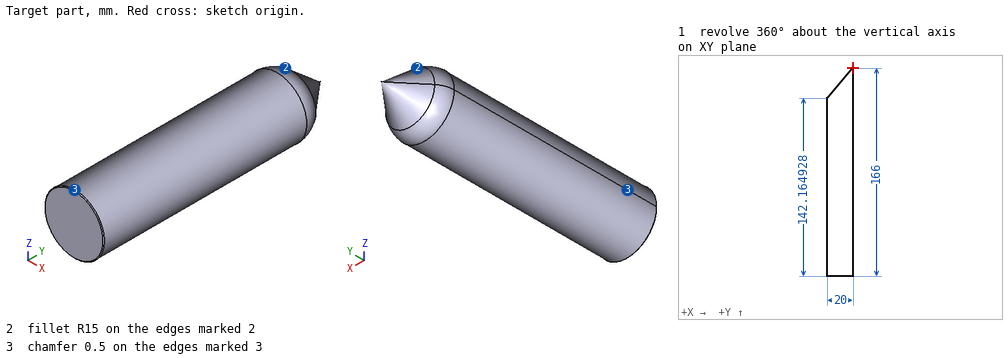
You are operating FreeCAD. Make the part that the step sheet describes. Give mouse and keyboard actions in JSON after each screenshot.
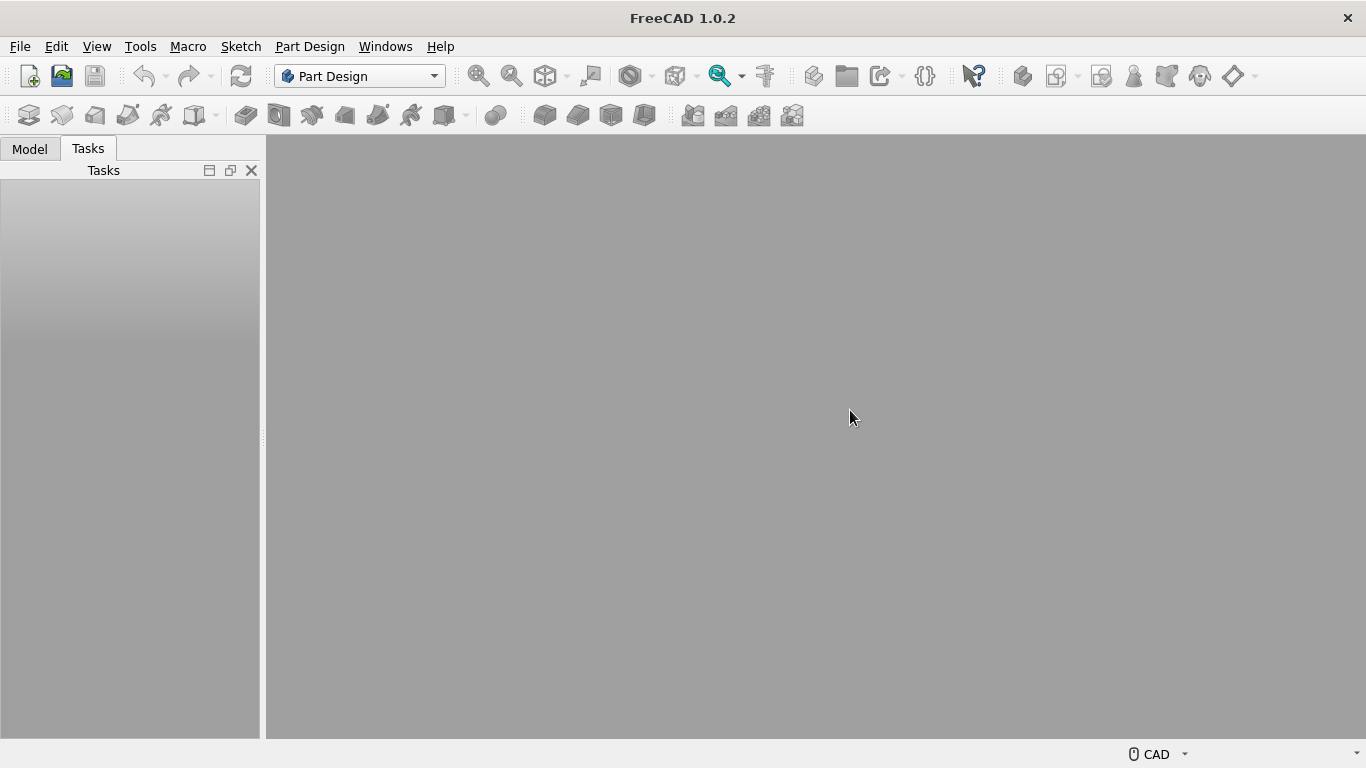
{"action": "key", "text": "ctrl+n"}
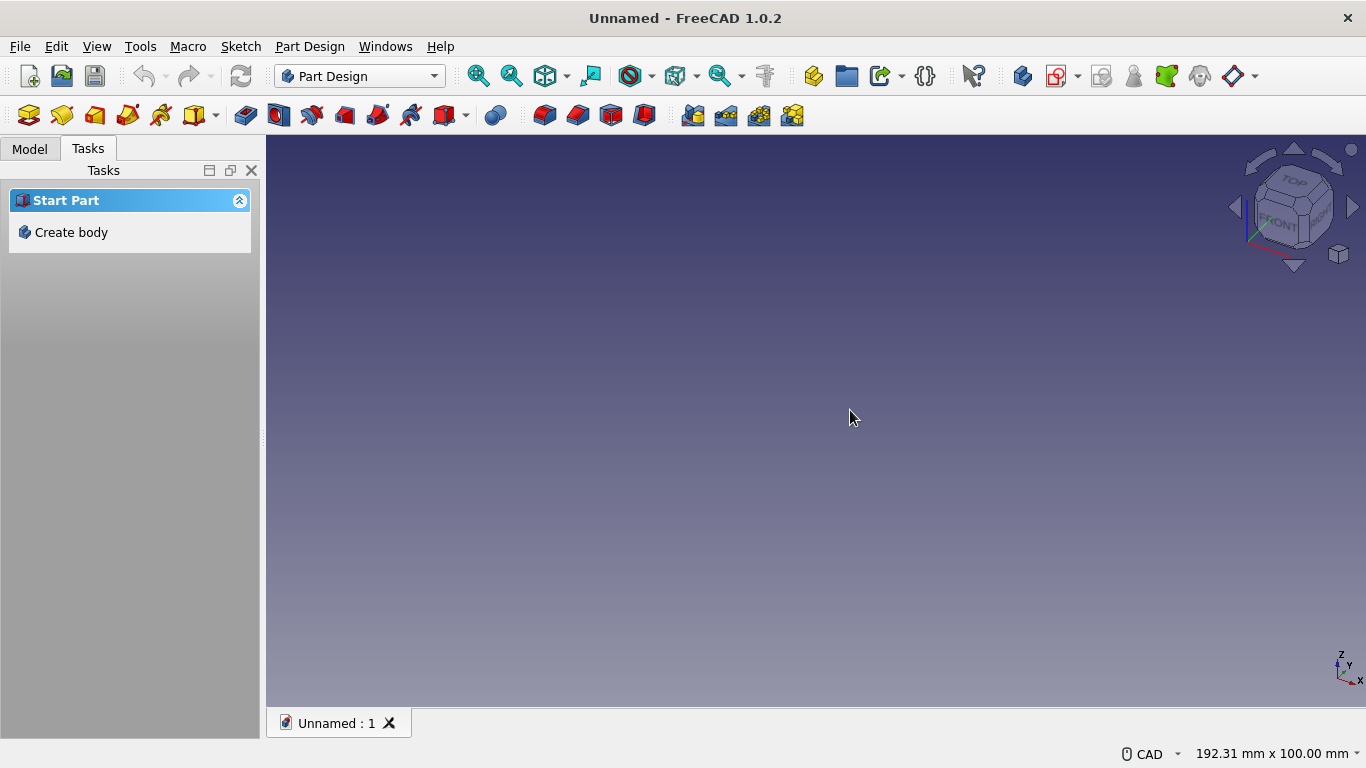
{"action": "left_click", "coordinate": [1056, 76]}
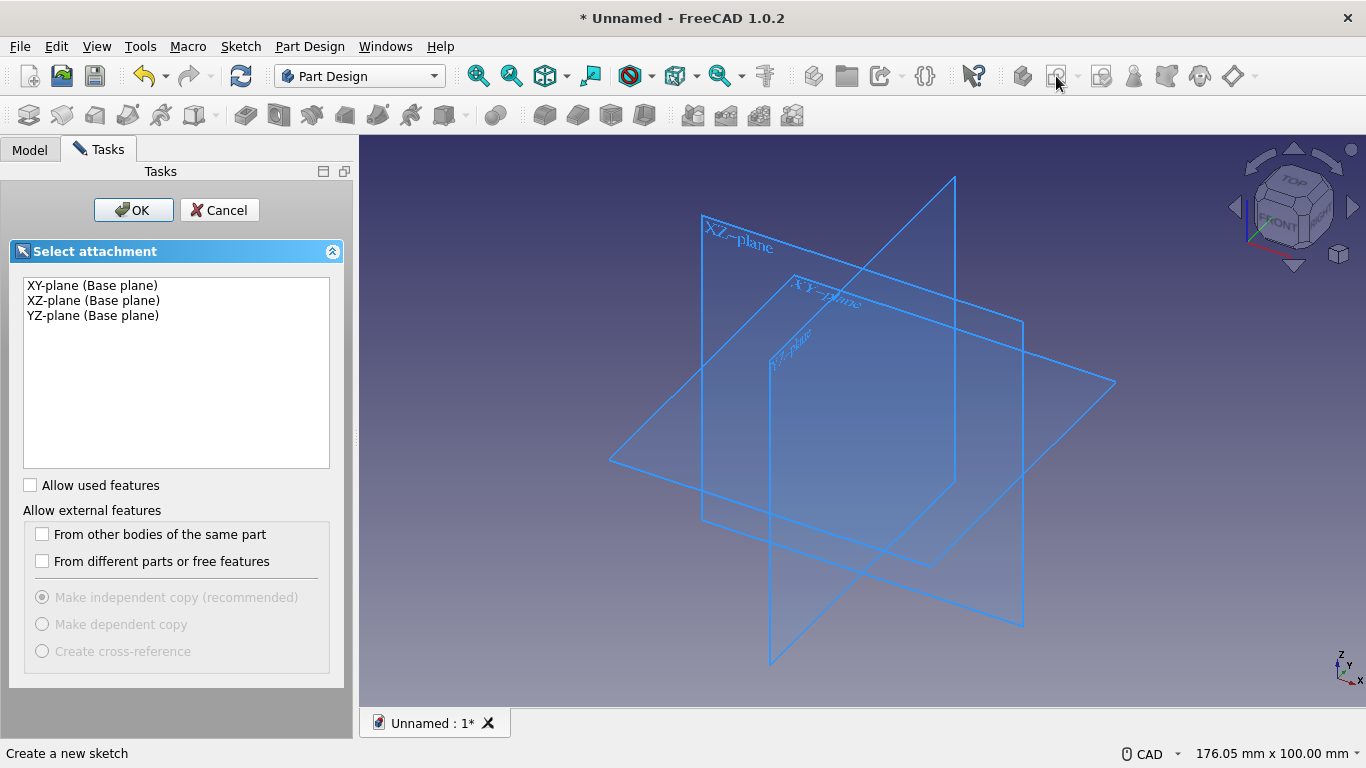
{"action": "left_click", "coordinate": [84, 286]}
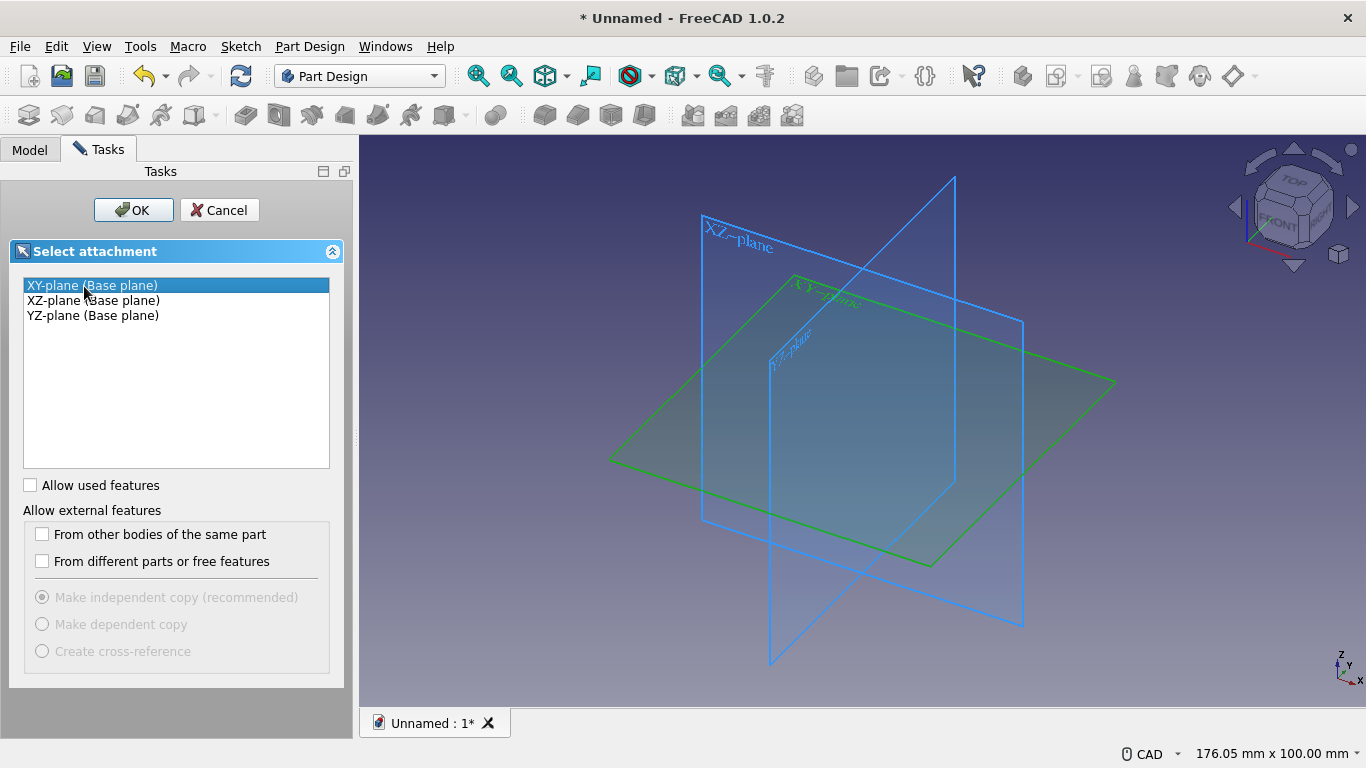
{"action": "left_click", "coordinate": [134, 210]}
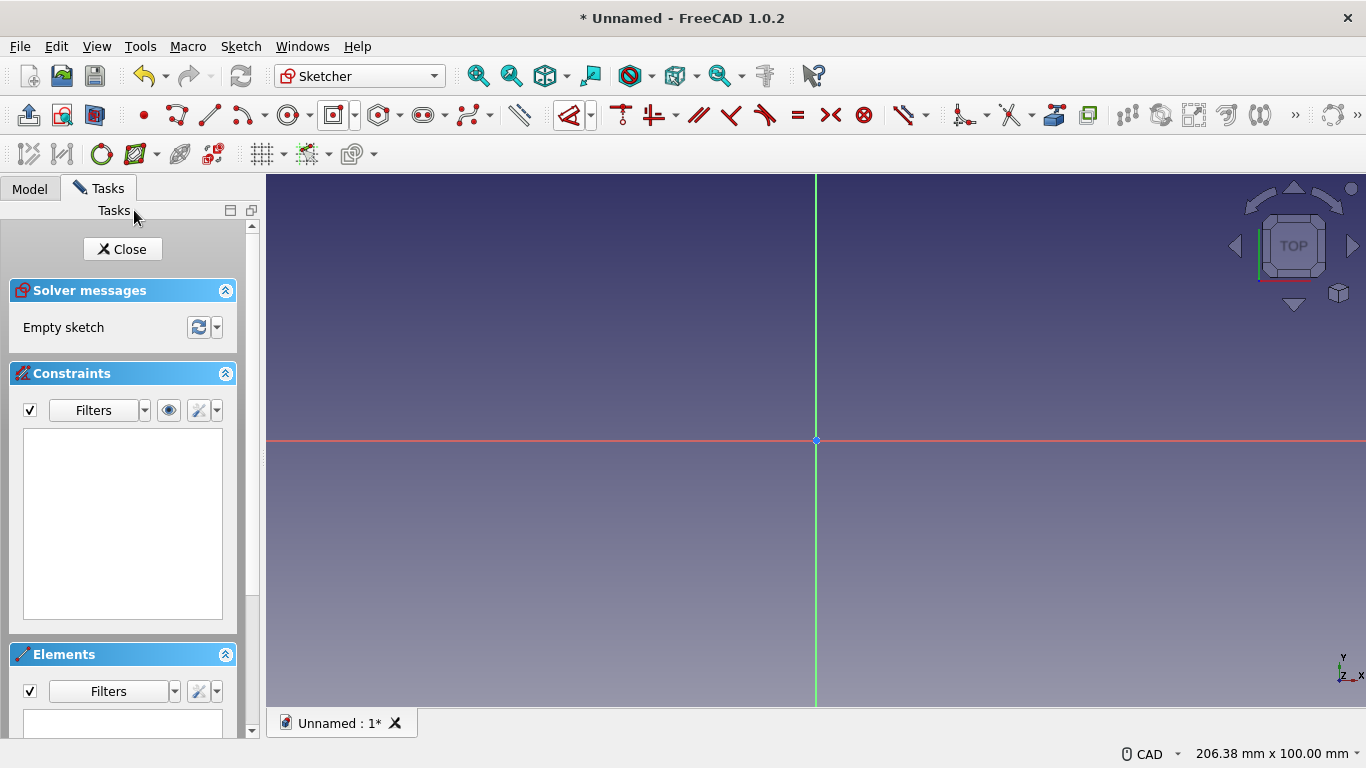
{"action": "scroll", "coordinate": [739, 202], "scroll_direction": "down", "scroll_amount": 5}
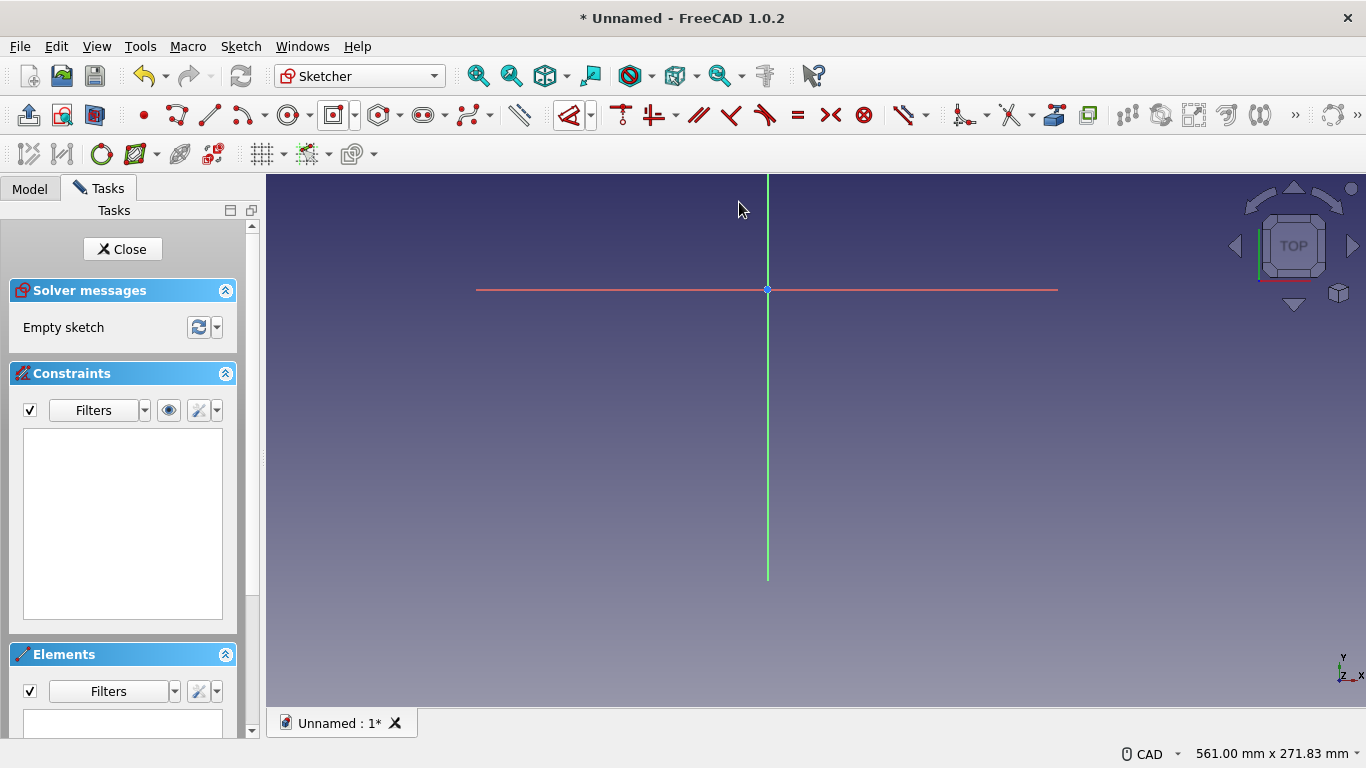
{"action": "key", "text": "g m"}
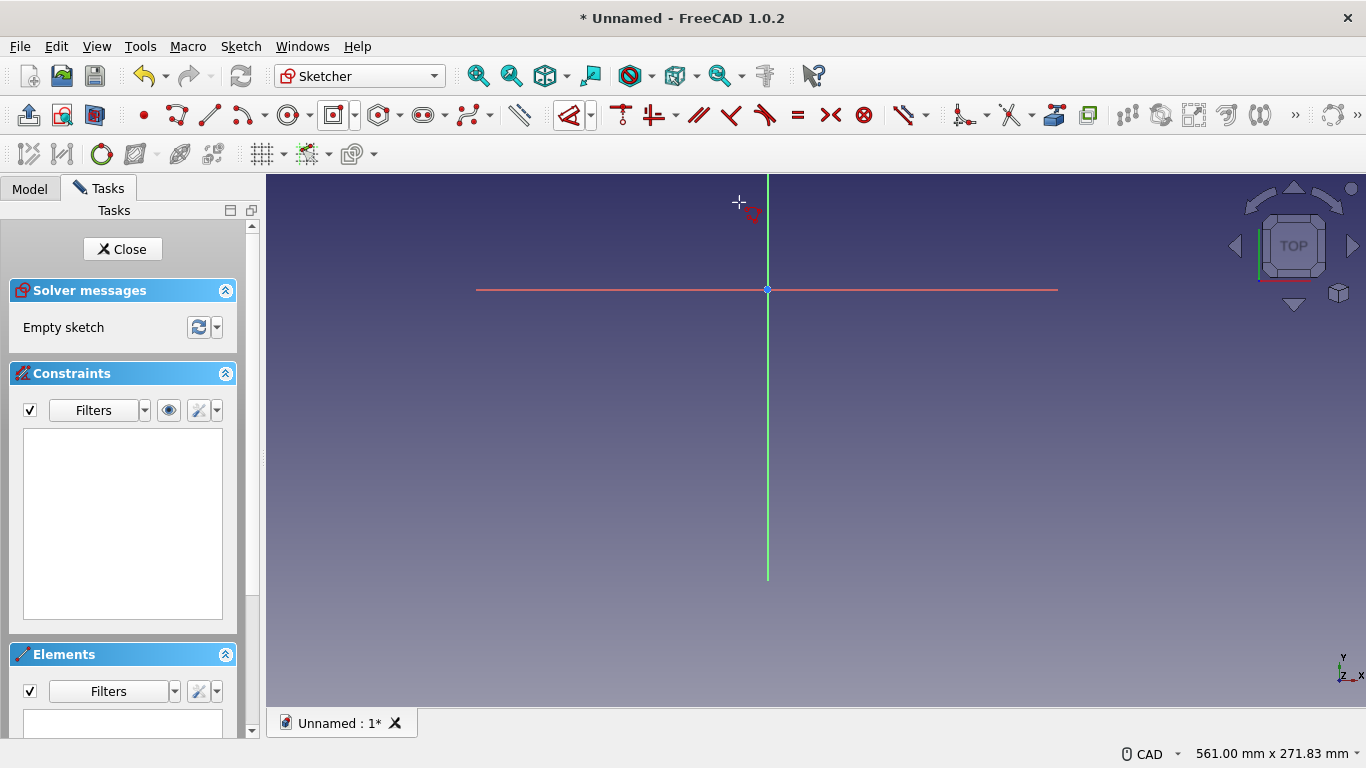
{"action": "left_click", "coordinate": [768, 290]}
{"action": "left_click", "coordinate": [728, 337]}
{"action": "left_click", "coordinate": [728, 615]}
{"action": "left_click", "coordinate": [759, 615]}
{"action": "left_click", "coordinate": [768, 290]}
{"action": "key", "text": "Escape"}
{"action": "key", "text": "Escape"}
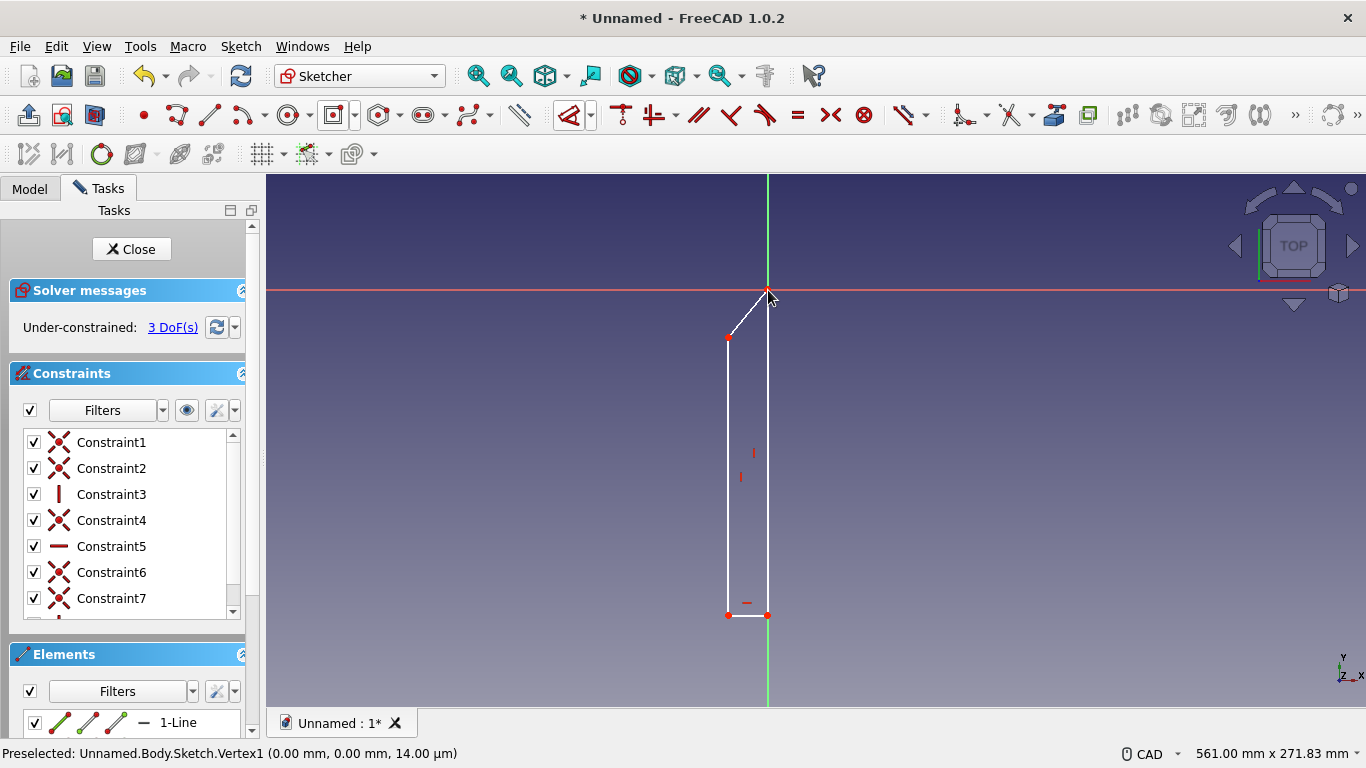
{"action": "left_click", "coordinate": [740, 616]}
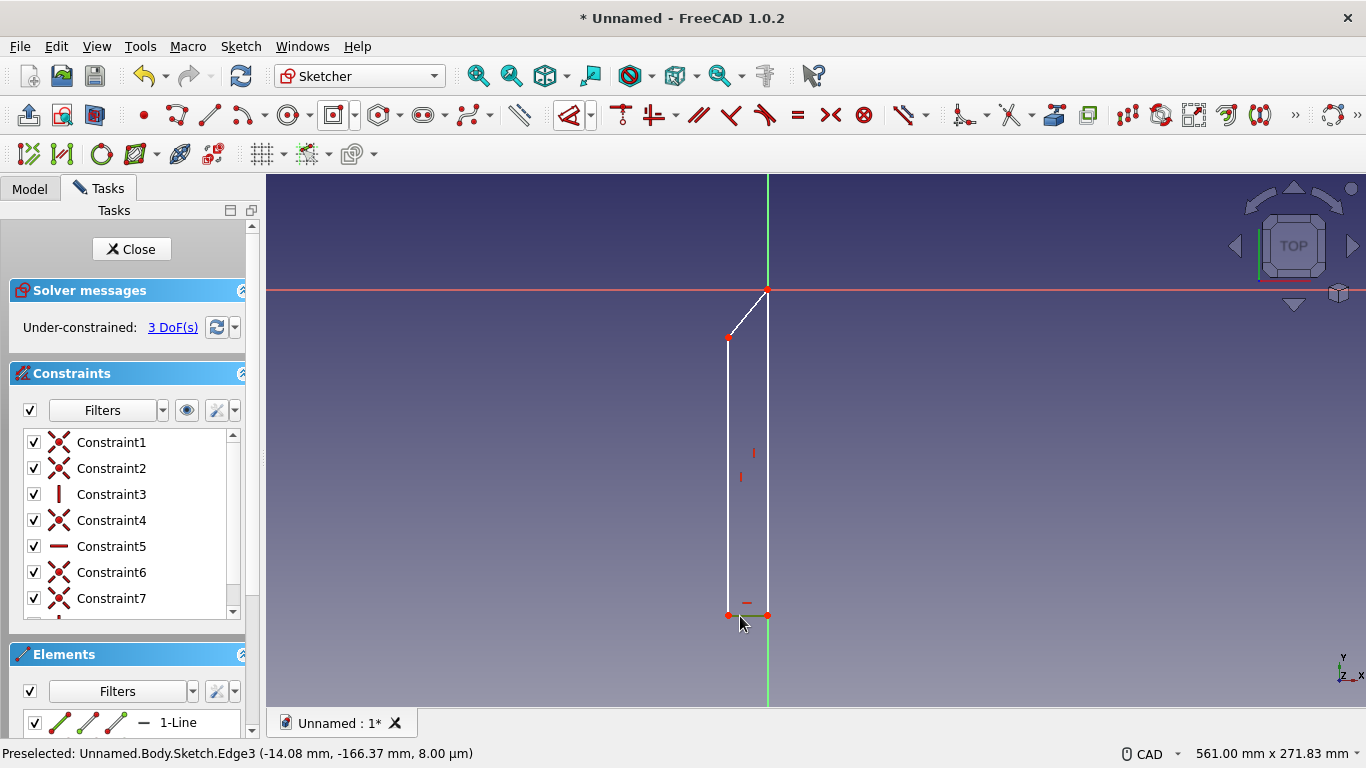
{"action": "key", "text": "l"}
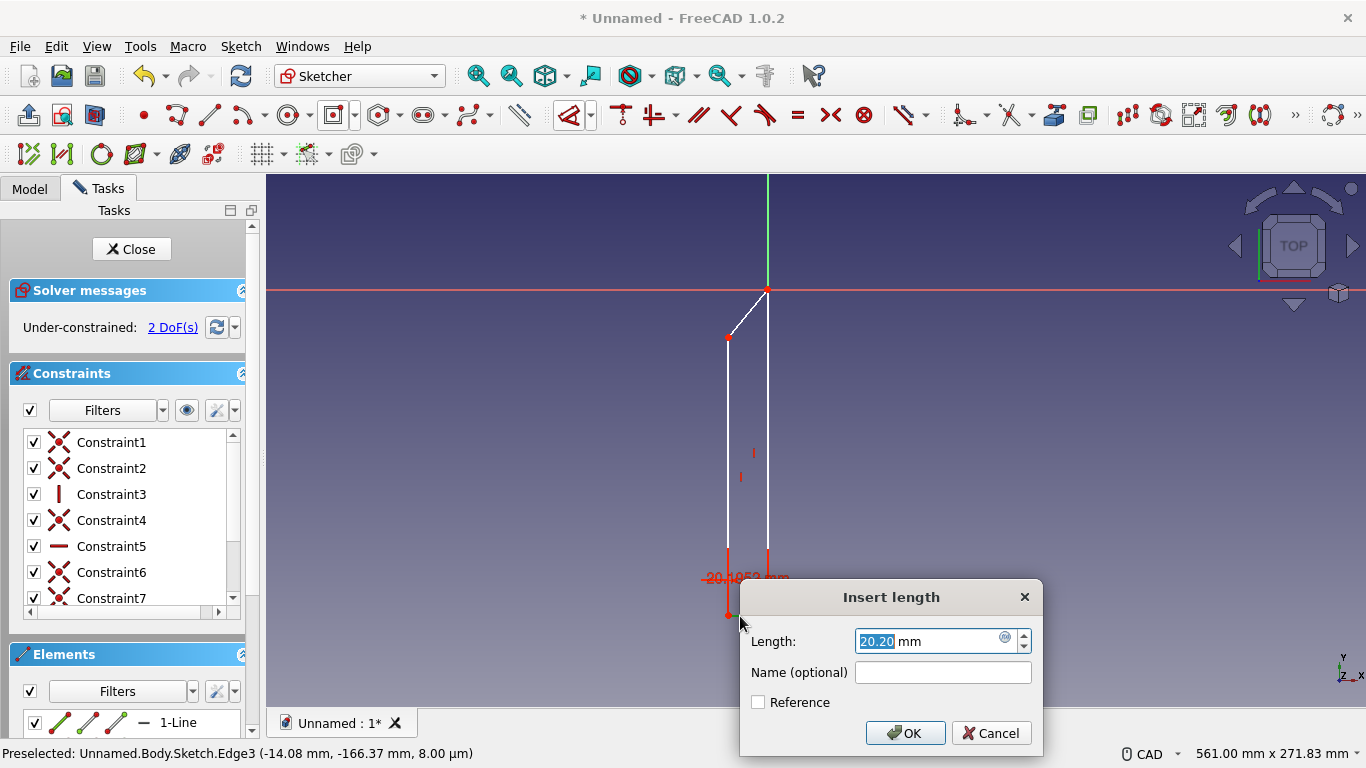
{"action": "type", "text": "20"}
{"action": "key", "text": "Return"}